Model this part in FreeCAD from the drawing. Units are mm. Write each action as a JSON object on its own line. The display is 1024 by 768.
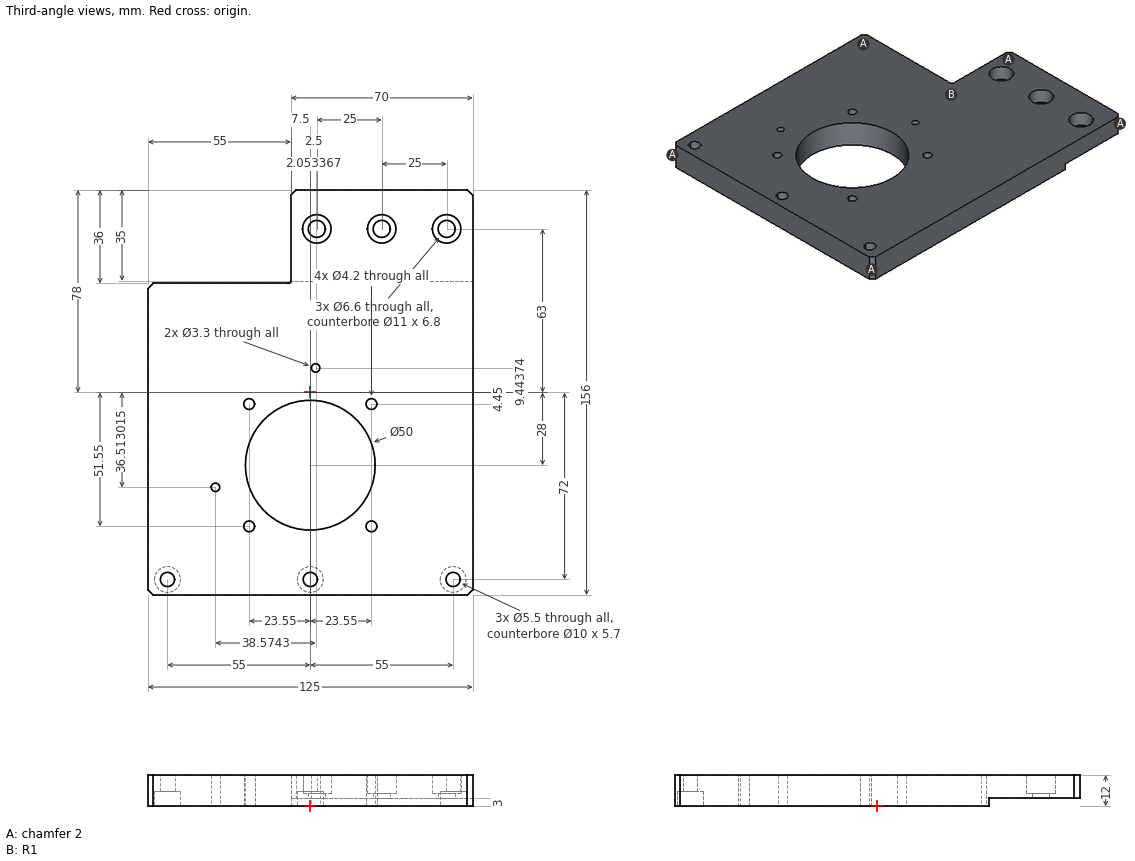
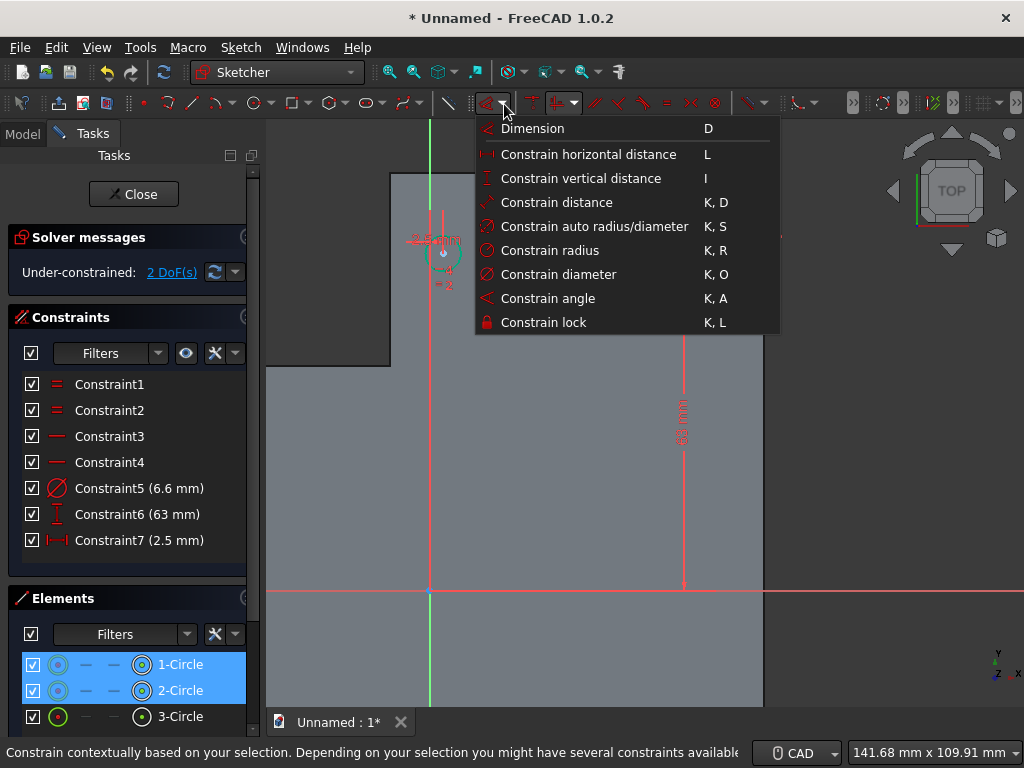
{"action": "left_click", "coordinate": [628, 154]}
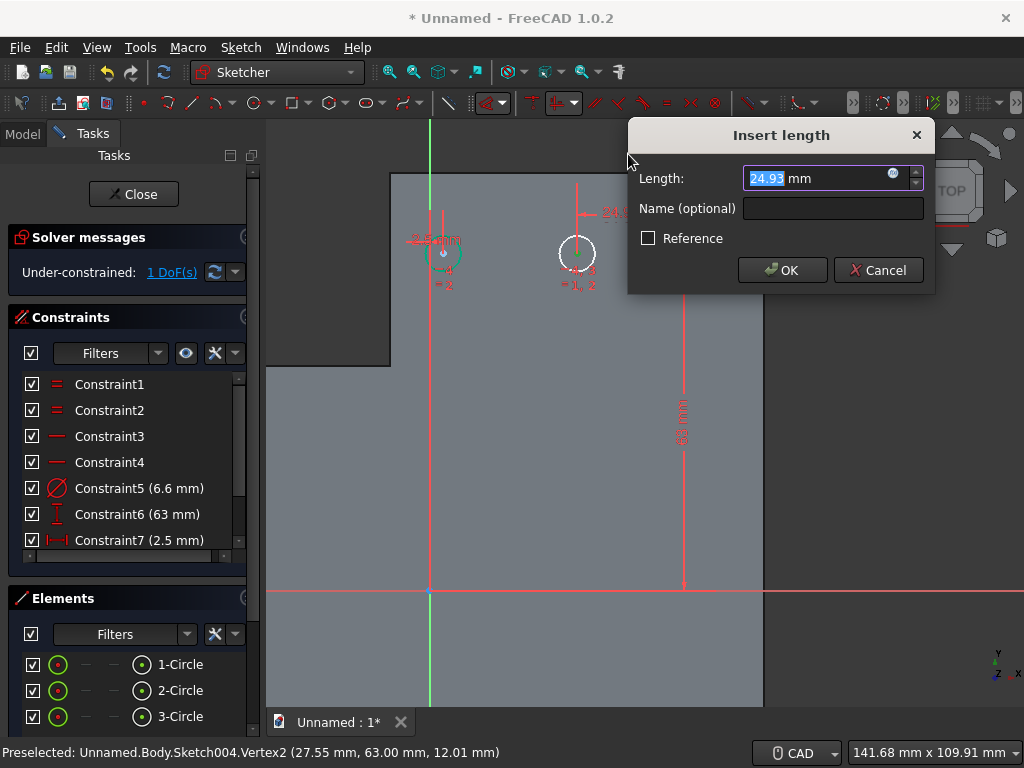
{"action": "type", "text": "25"}
{"action": "key", "text": "Return"}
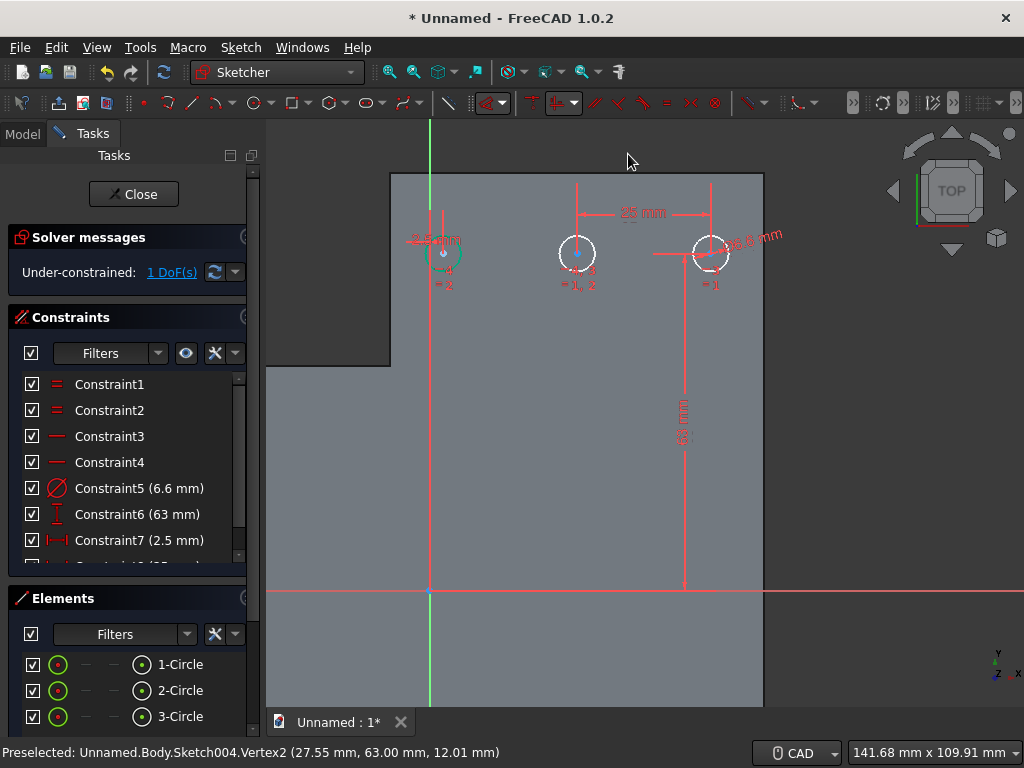
{"action": "left_click", "coordinate": [577, 254]}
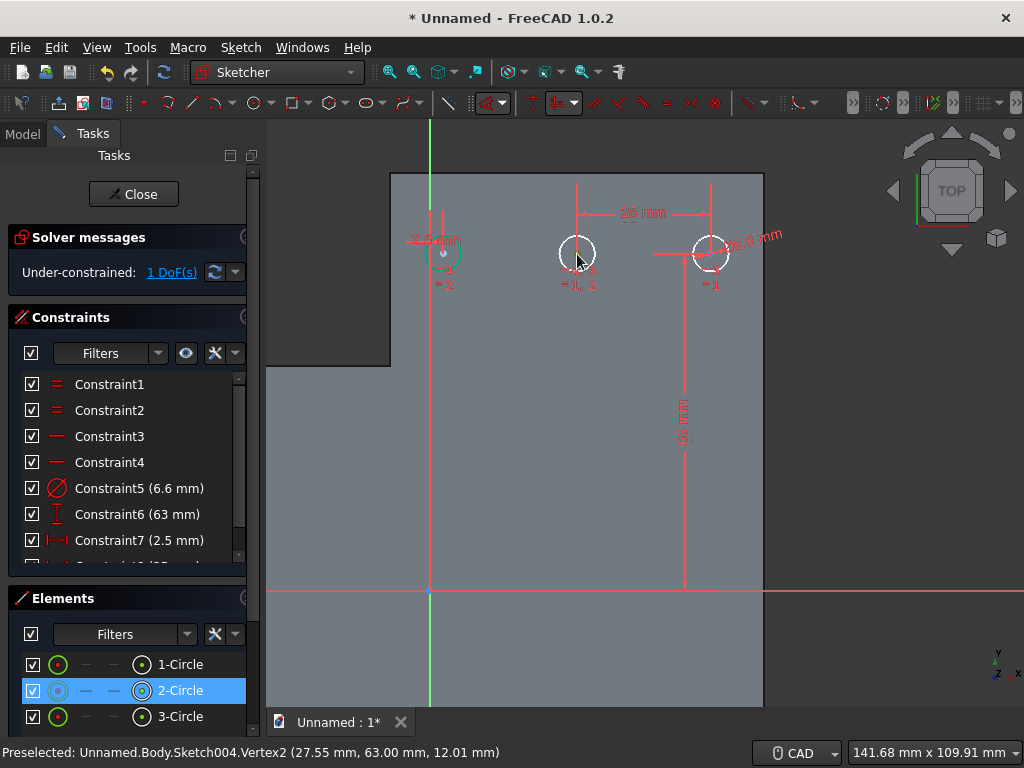
{"action": "left_click", "coordinate": [443, 254]}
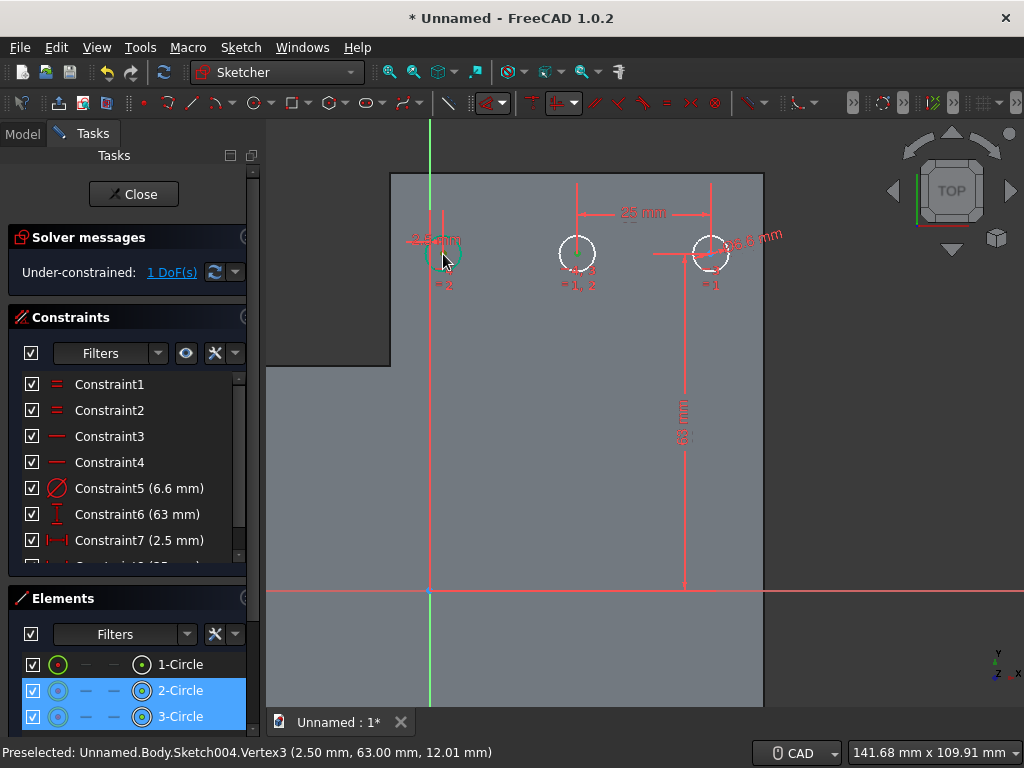
{"action": "left_click", "coordinate": [504, 104]}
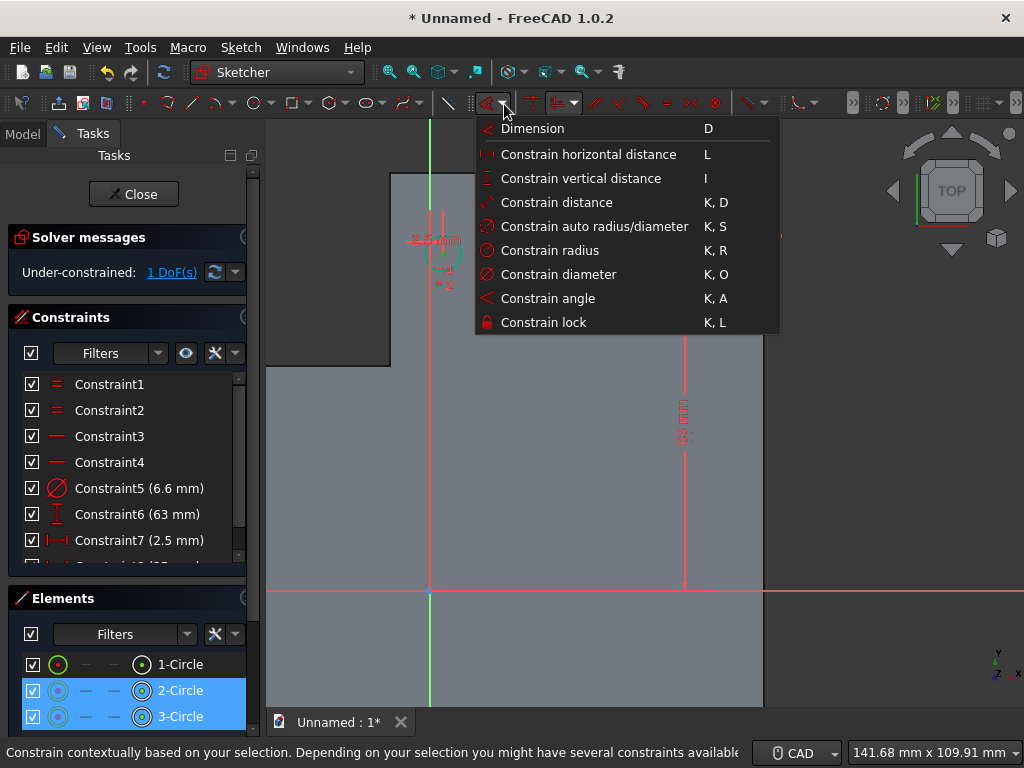
{"action": "left_click", "coordinate": [628, 154]}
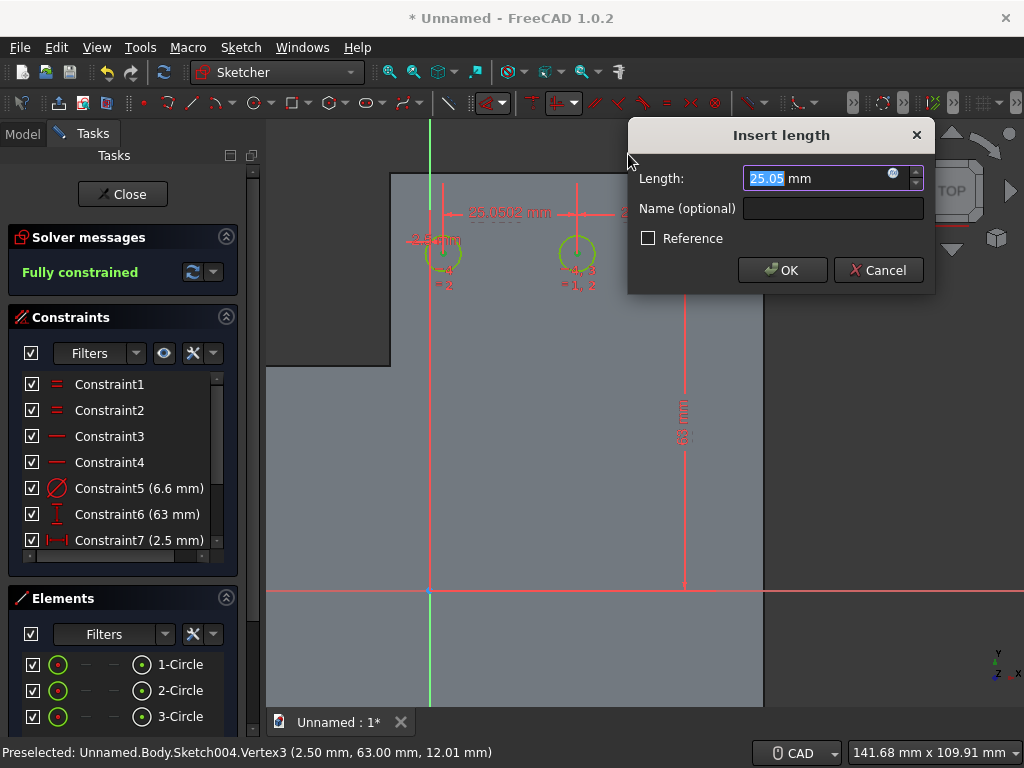
{"action": "type", "text": "25"}
{"action": "key", "text": "Return"}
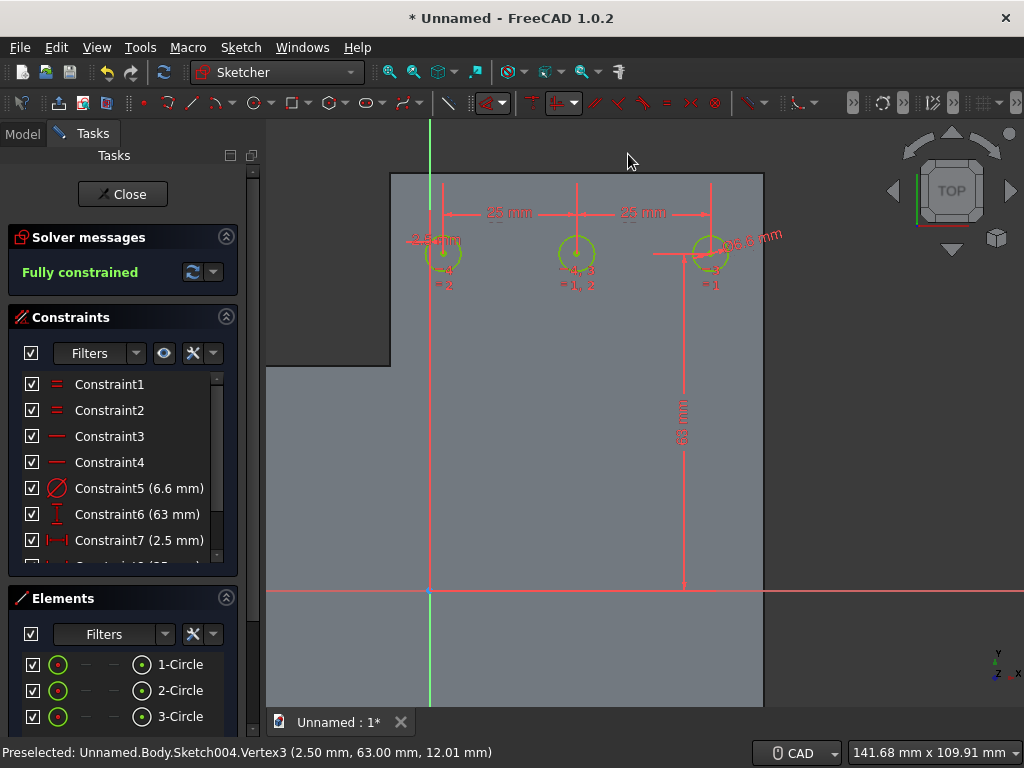
{"action": "left_click", "coordinate": [123, 194]}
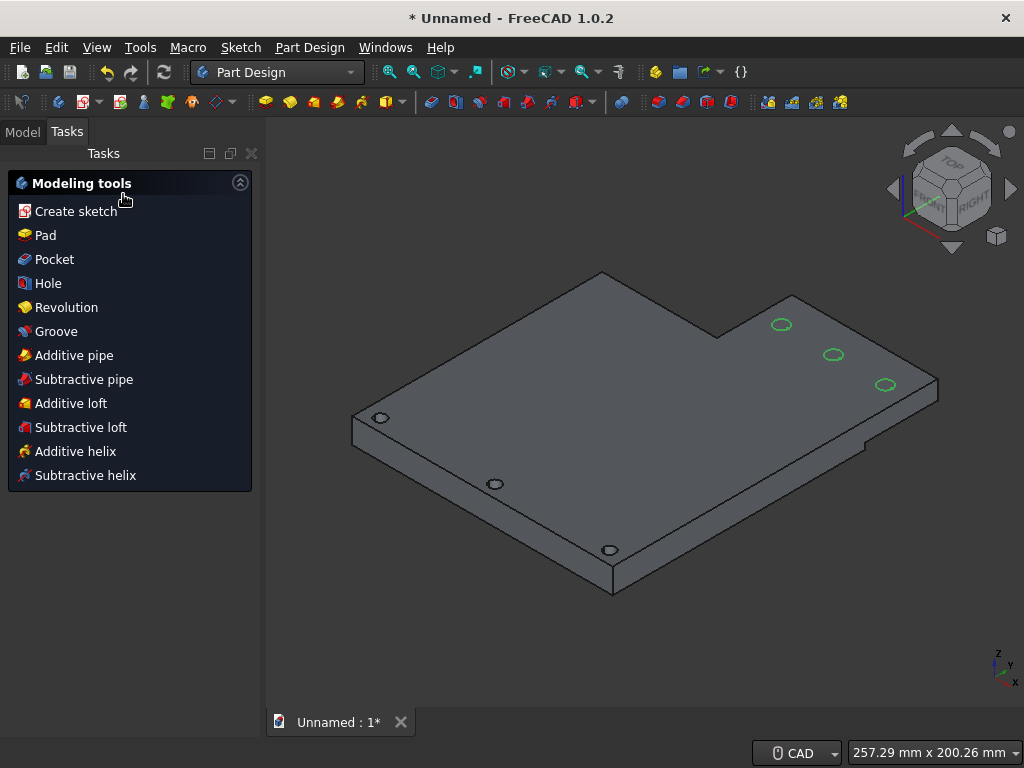
{"action": "left_click", "coordinate": [456, 102]}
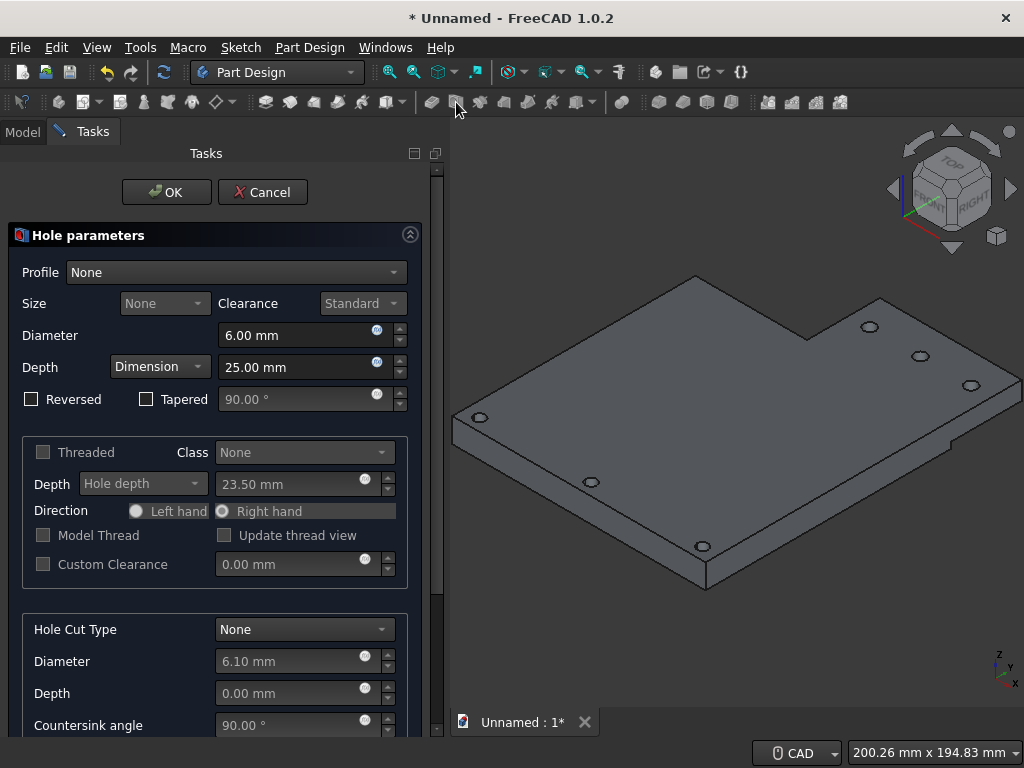
{"action": "triple_click", "coordinate": [305, 335]}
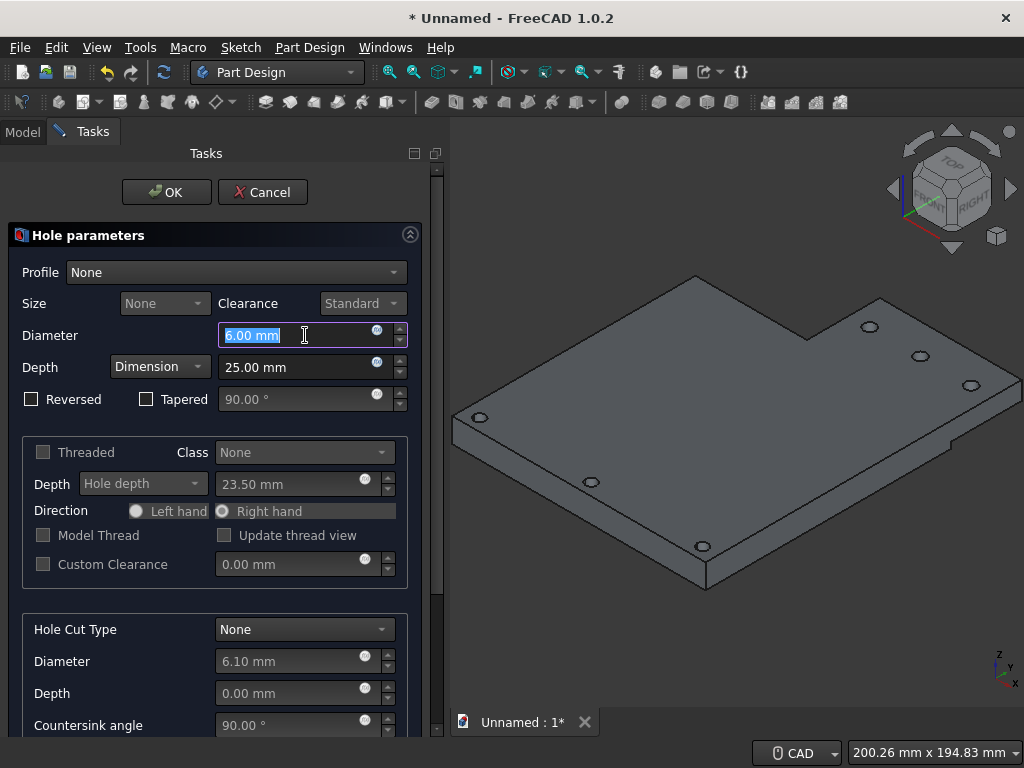
{"action": "type", "text": "6.6"}
{"action": "key", "text": "Tab"}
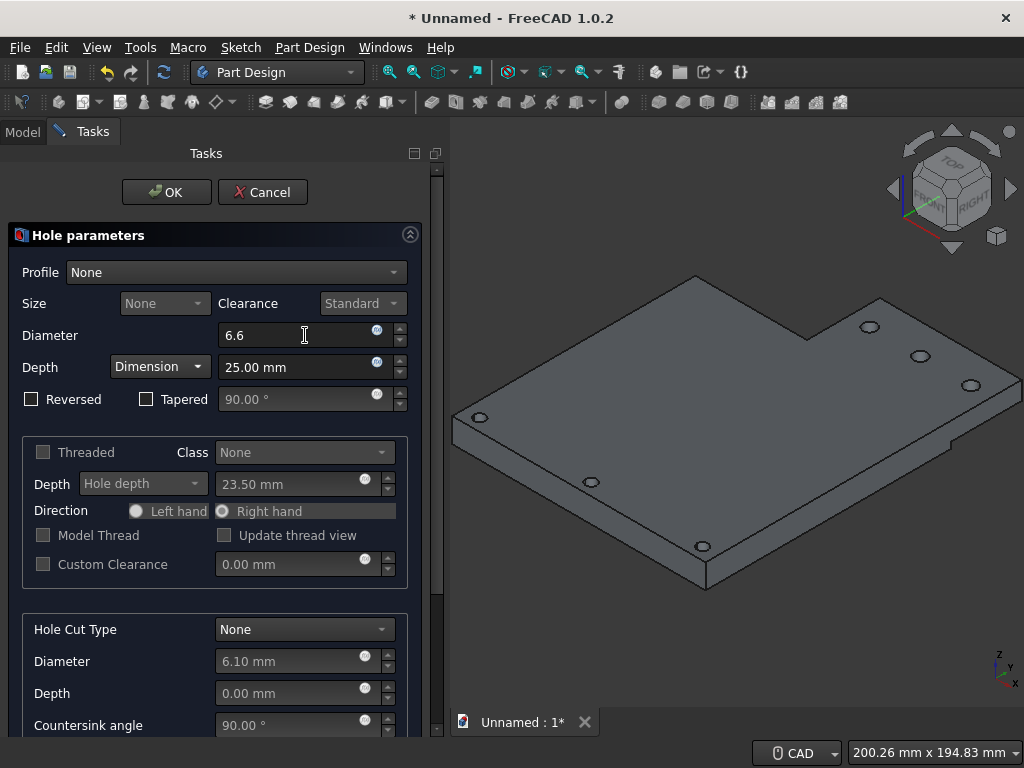
{"action": "left_click", "coordinate": [161, 366]}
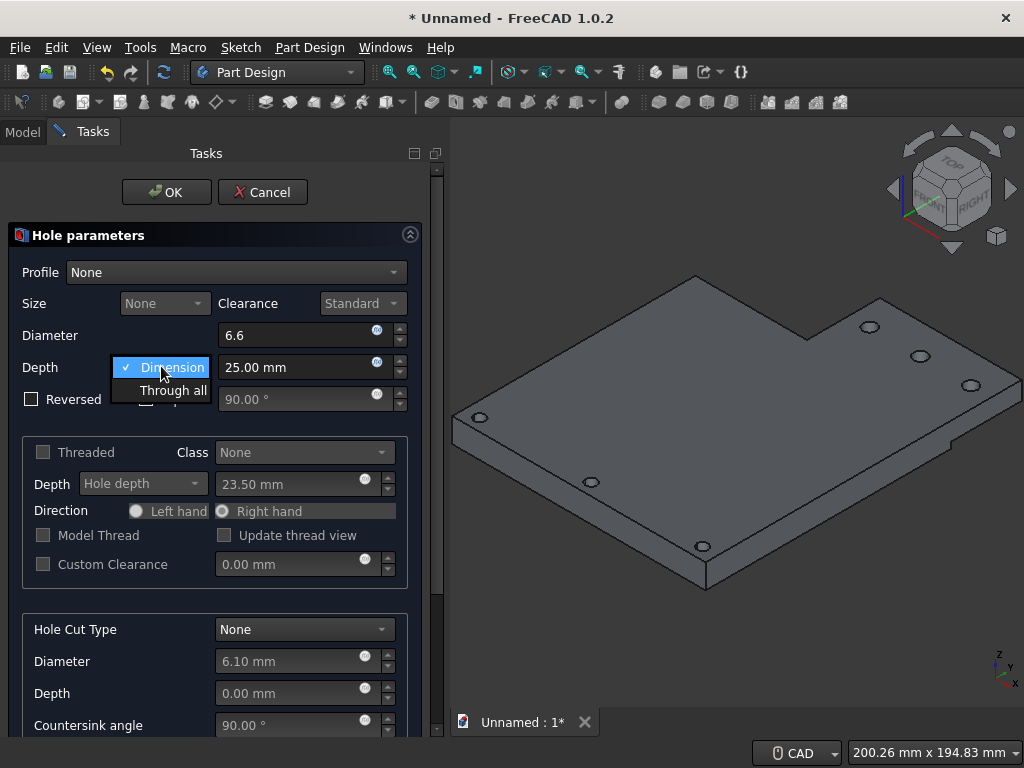
{"action": "left_click", "coordinate": [160, 390]}